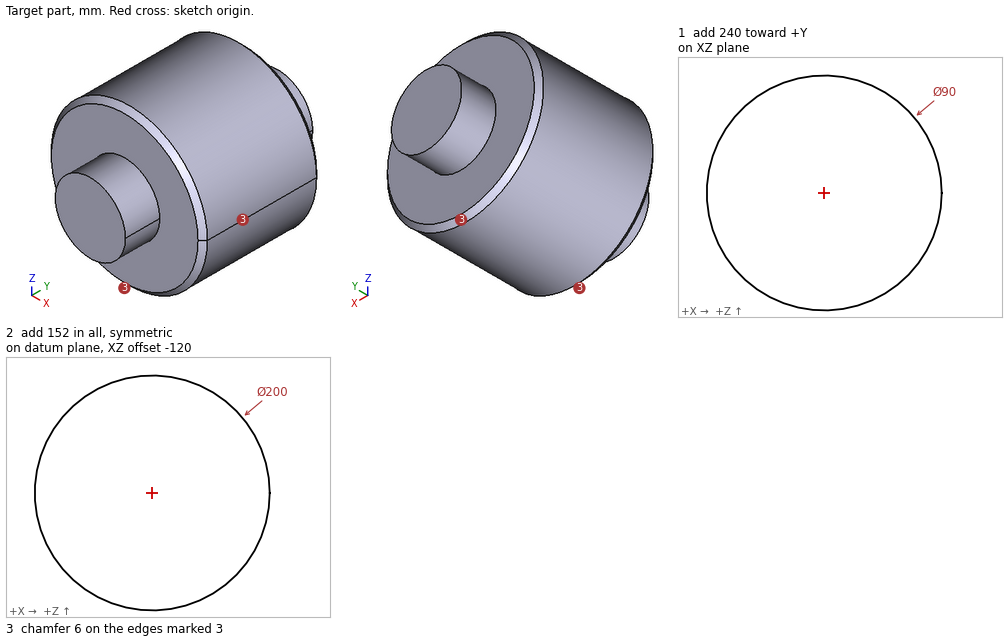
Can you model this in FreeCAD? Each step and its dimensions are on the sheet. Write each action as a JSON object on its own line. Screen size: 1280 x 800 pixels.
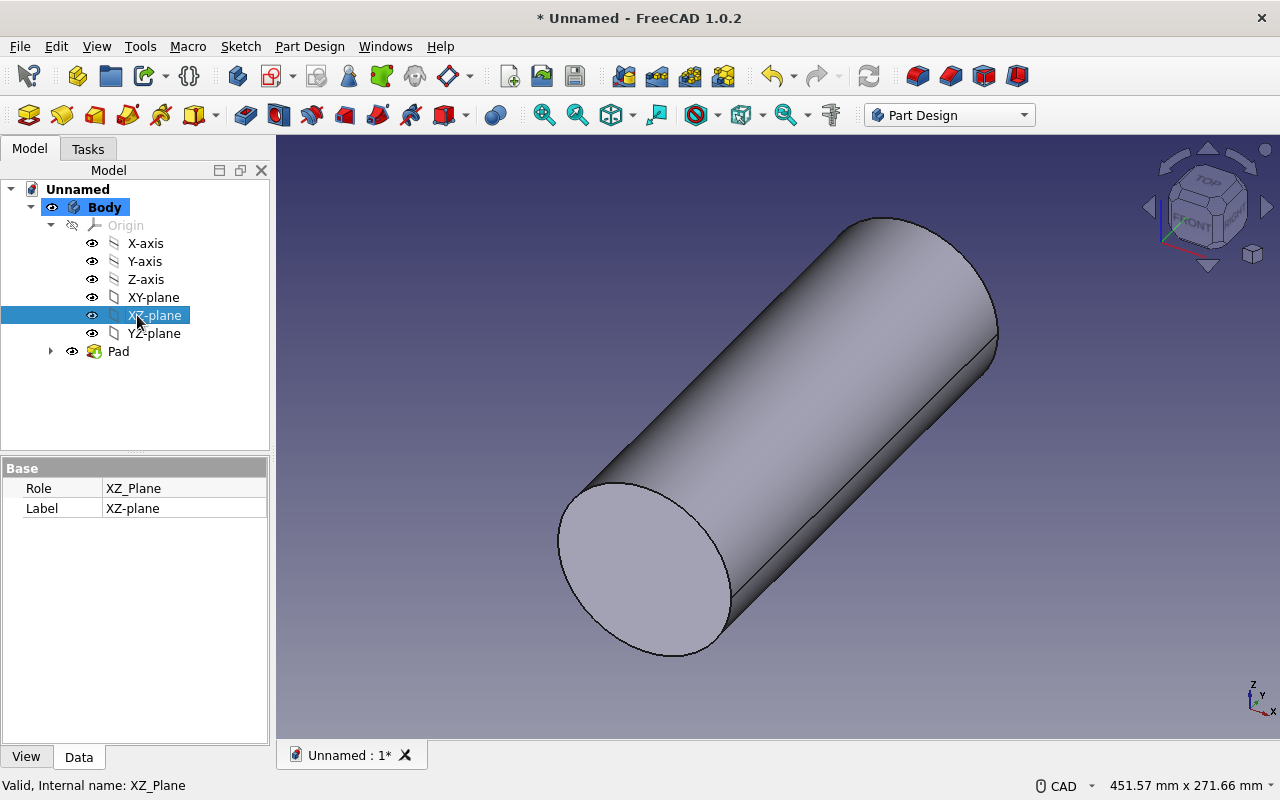
{"action": "left_click", "coordinate": [448, 76]}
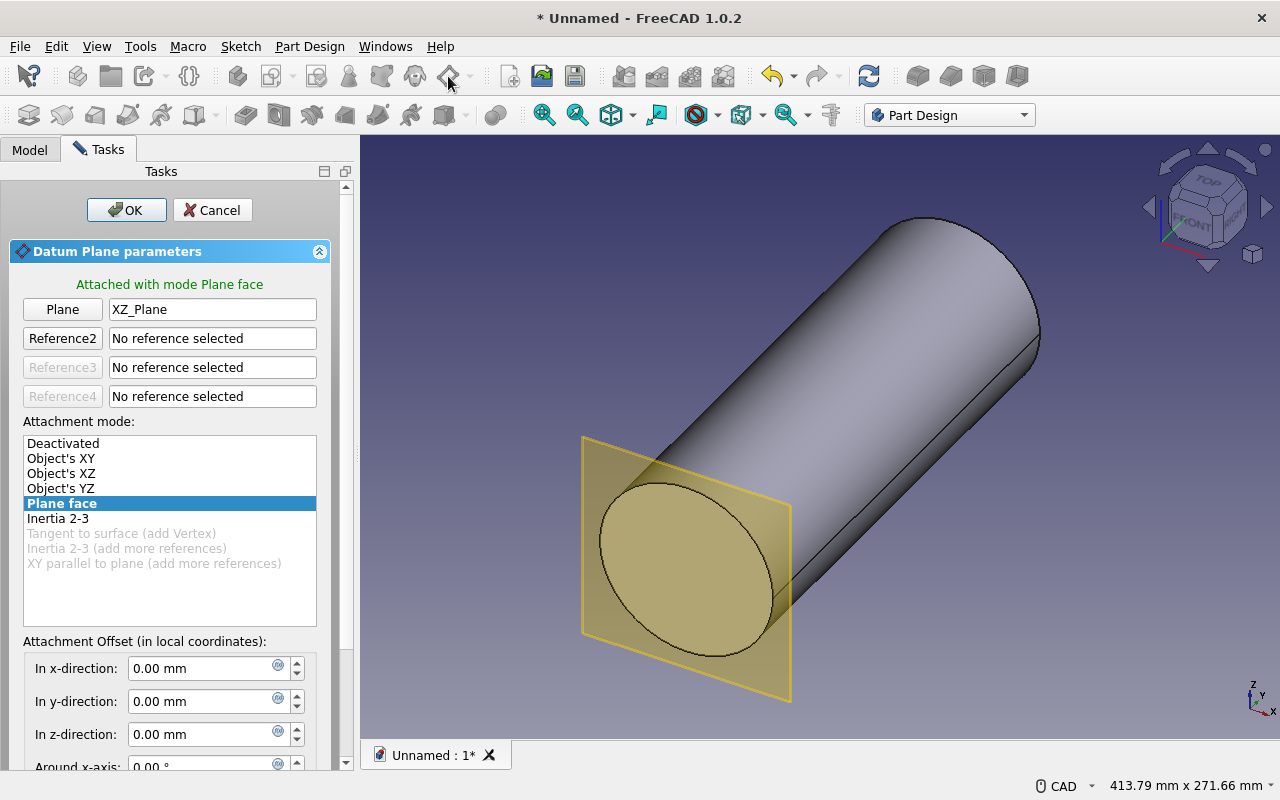
{"action": "triple_click", "coordinate": [210, 734]}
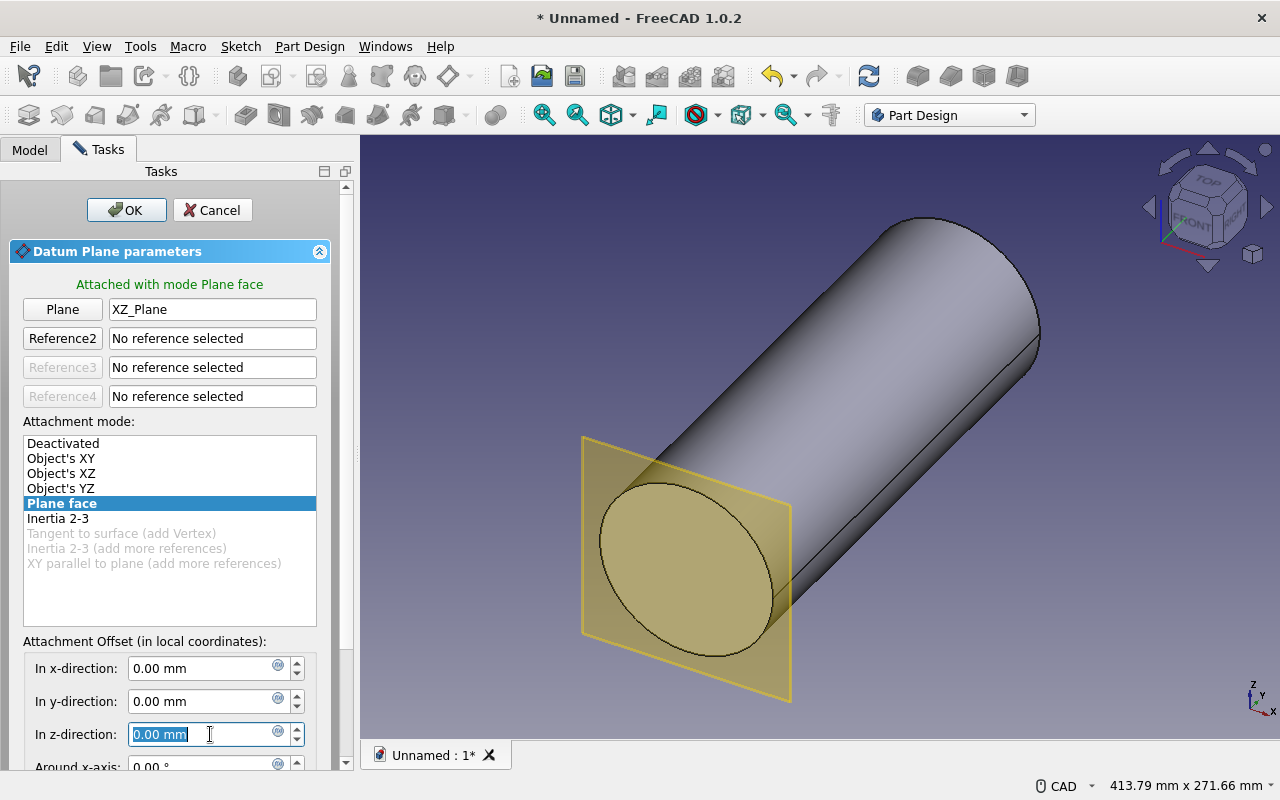
{"action": "type", "text": "-120"}
{"action": "key", "text": "Tab"}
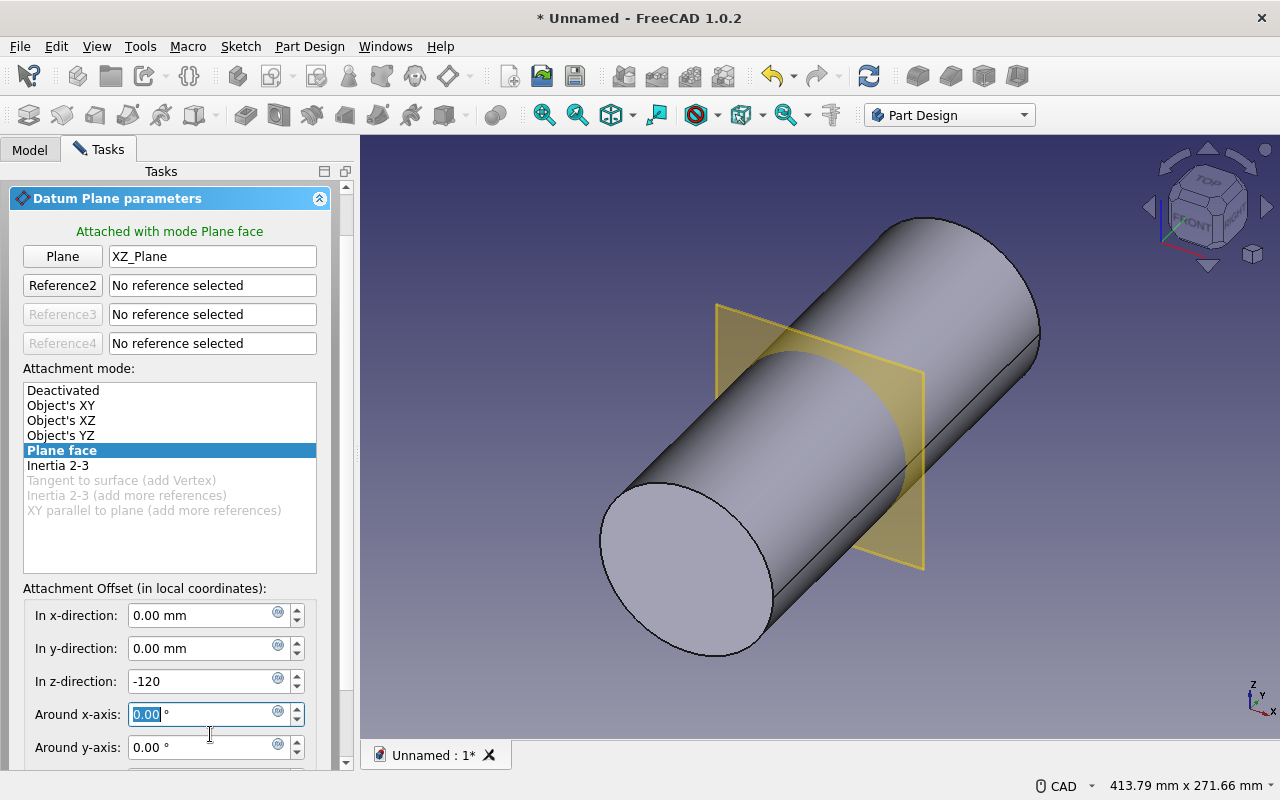
{"action": "scroll", "coordinate": [346, 476], "scroll_direction": "up", "scroll_amount": 2}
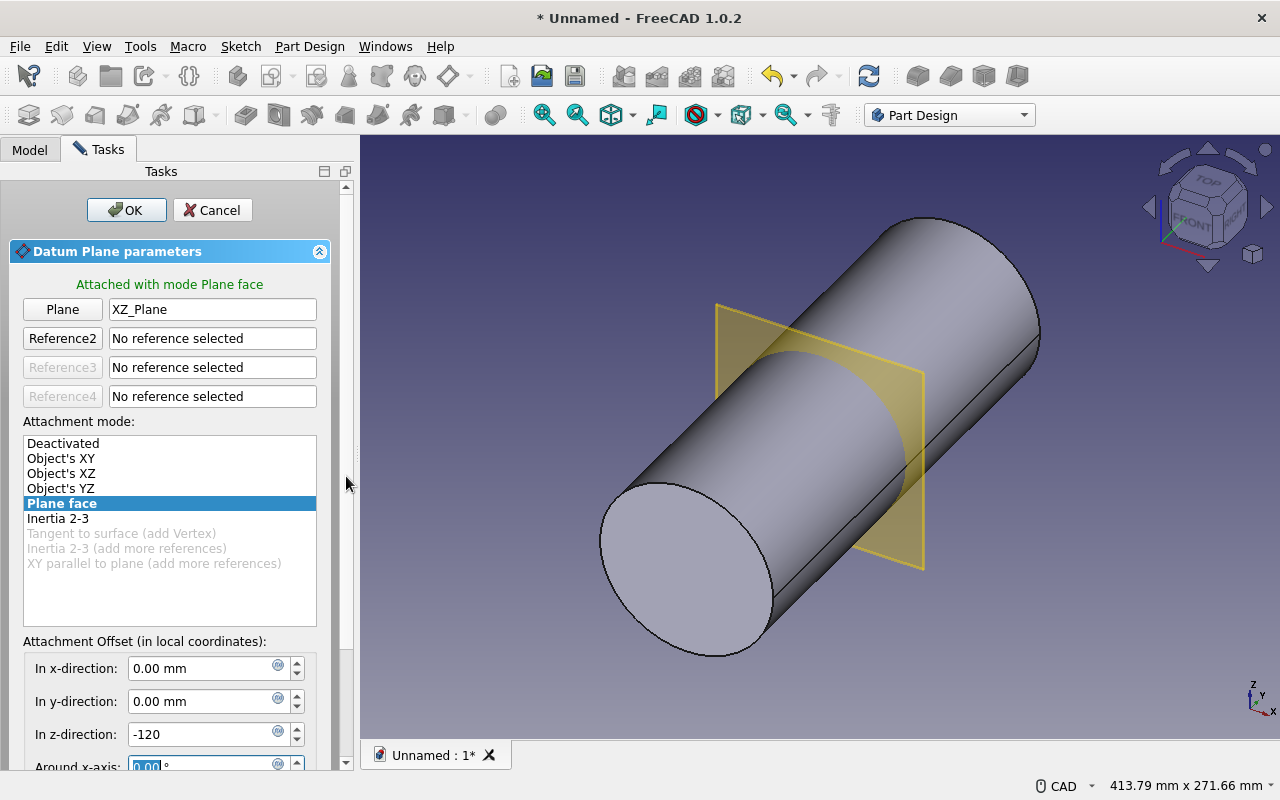
{"action": "left_click", "coordinate": [127, 210]}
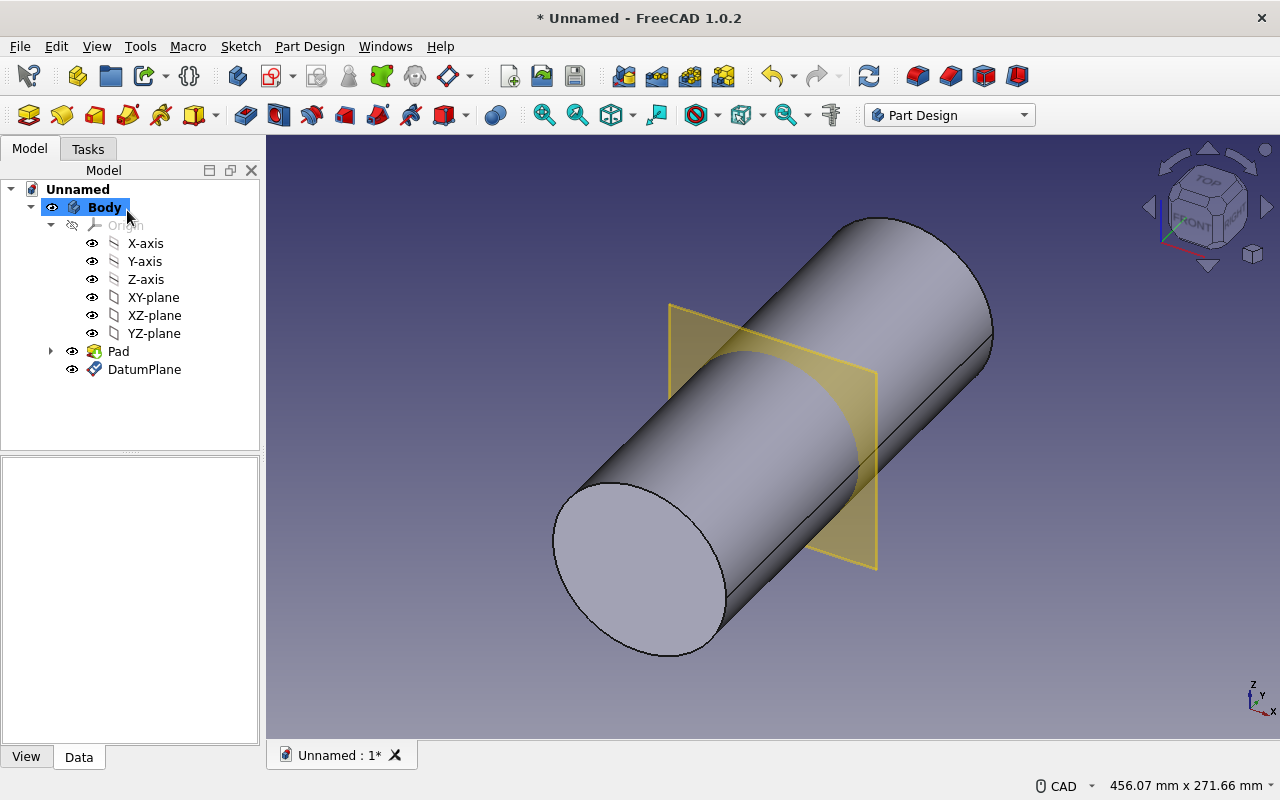
{"action": "left_click", "coordinate": [117, 369]}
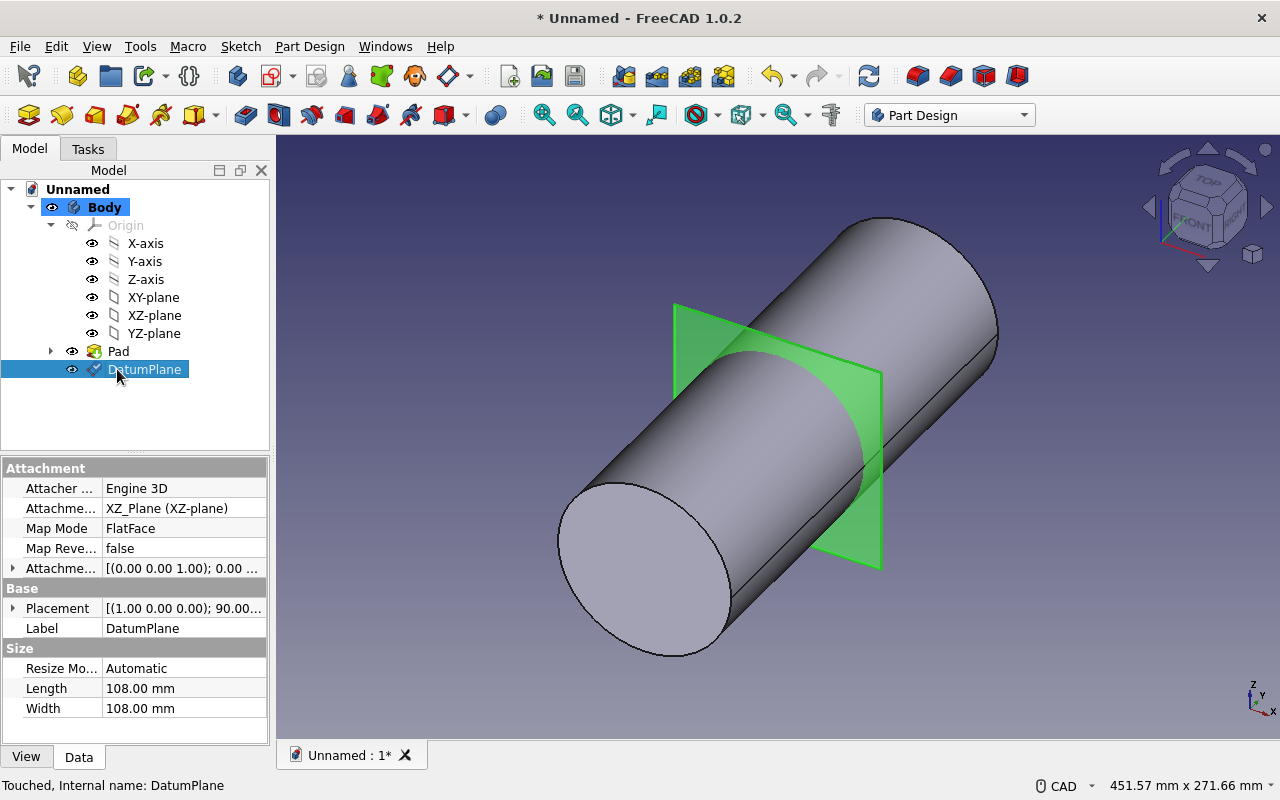
{"action": "left_click", "coordinate": [270, 76]}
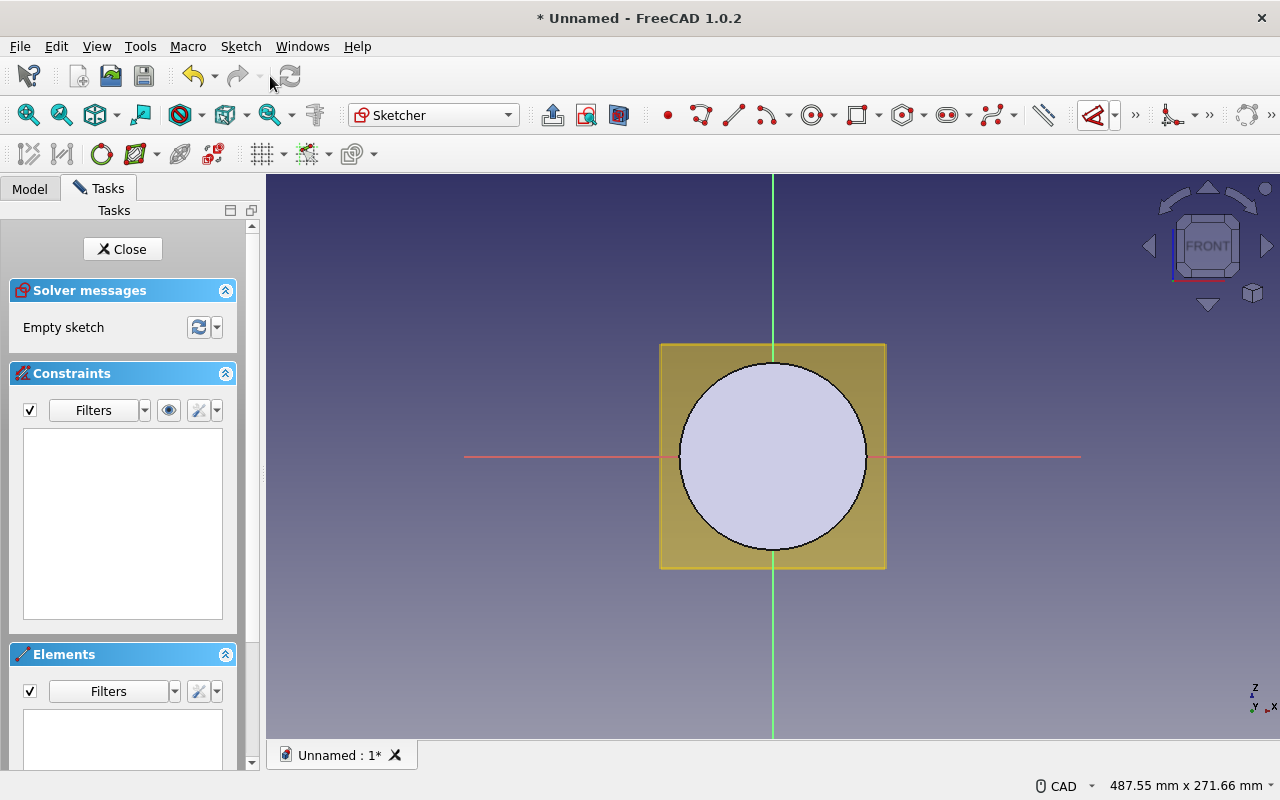
{"action": "left_click", "coordinate": [619, 116]}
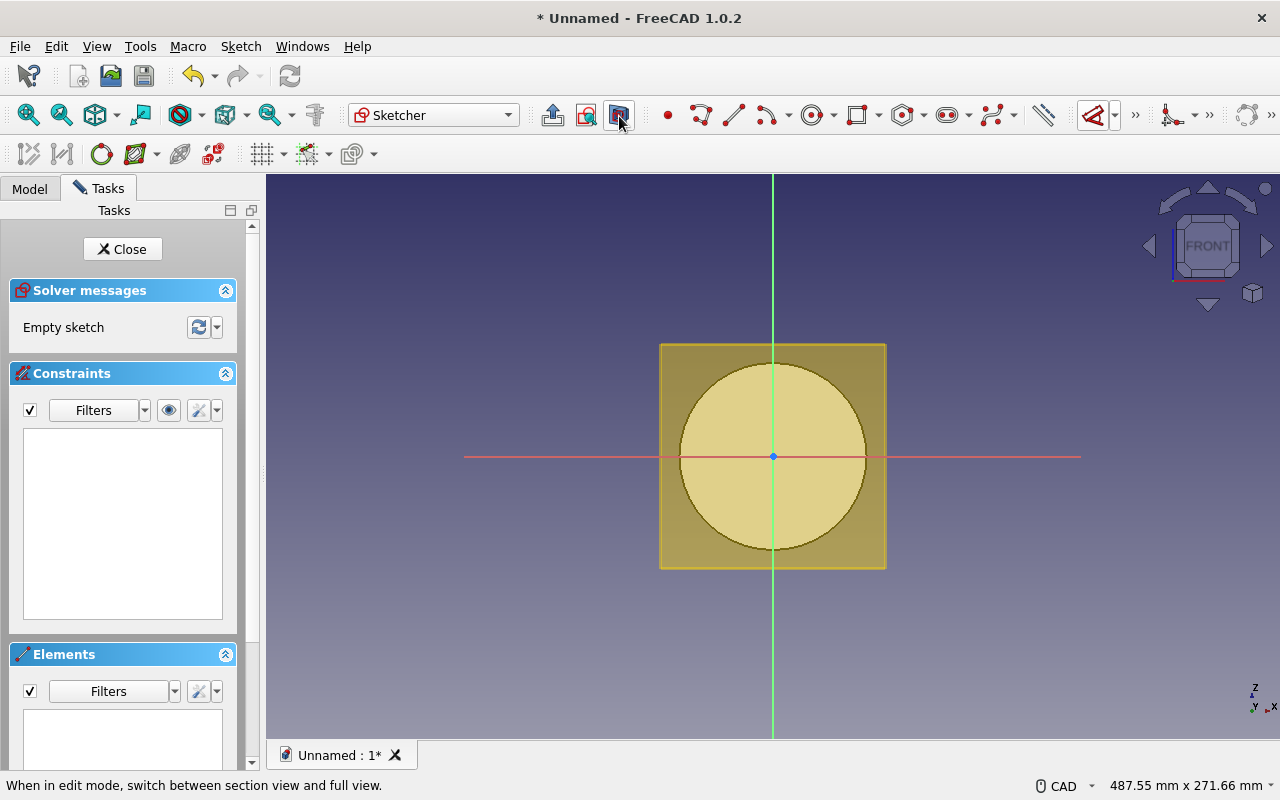
{"action": "key", "text": "g c"}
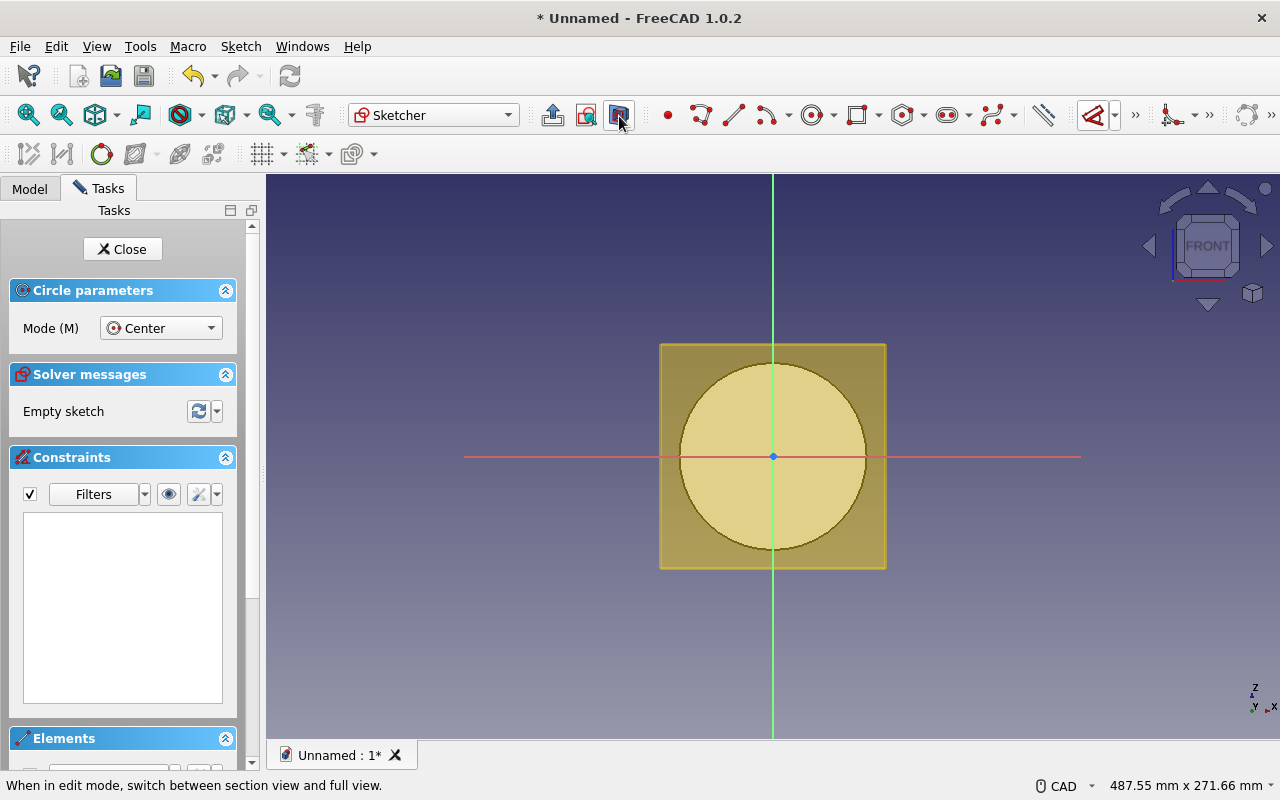
{"action": "left_click", "coordinate": [773, 457]}
{"action": "left_click", "coordinate": [920, 309]}
{"action": "key", "text": "Escape"}